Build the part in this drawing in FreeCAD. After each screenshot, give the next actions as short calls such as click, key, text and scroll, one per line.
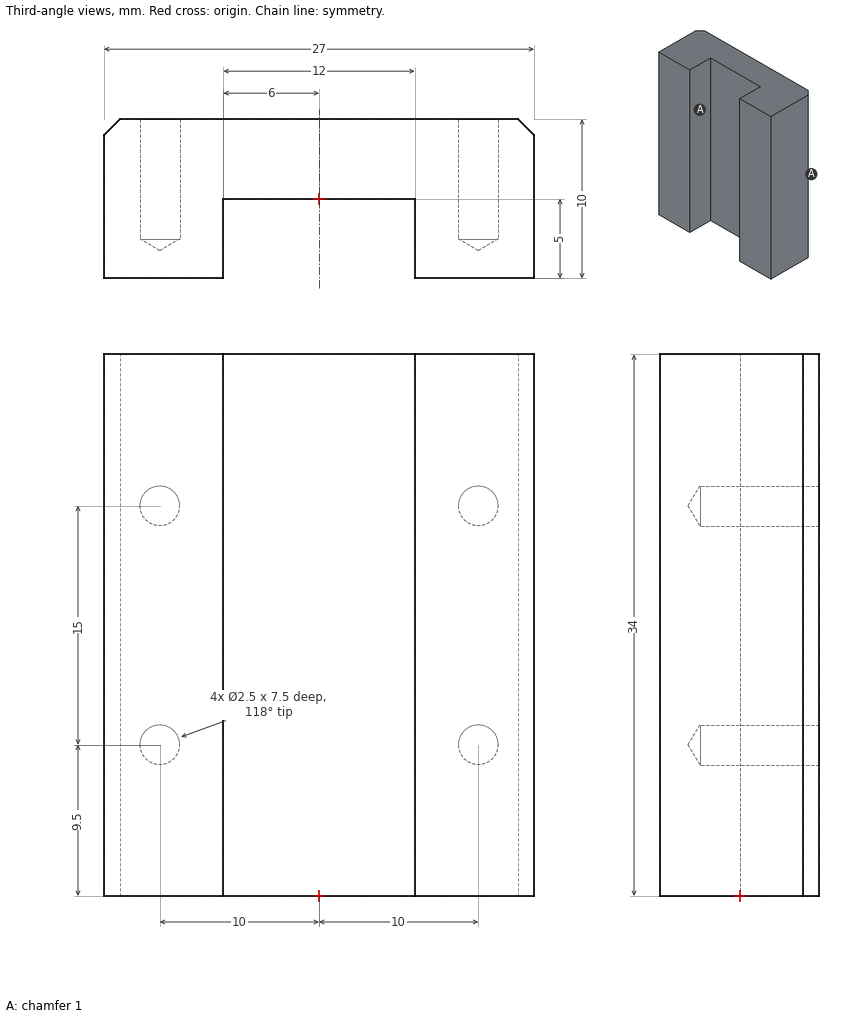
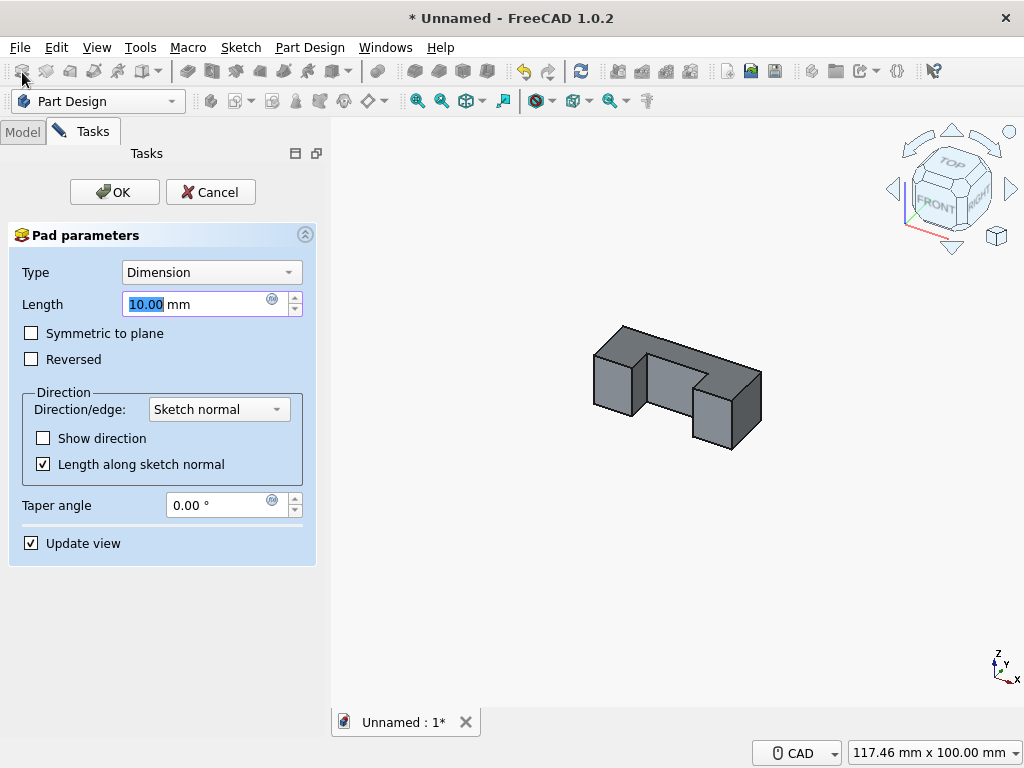
text(34)
key(Tab)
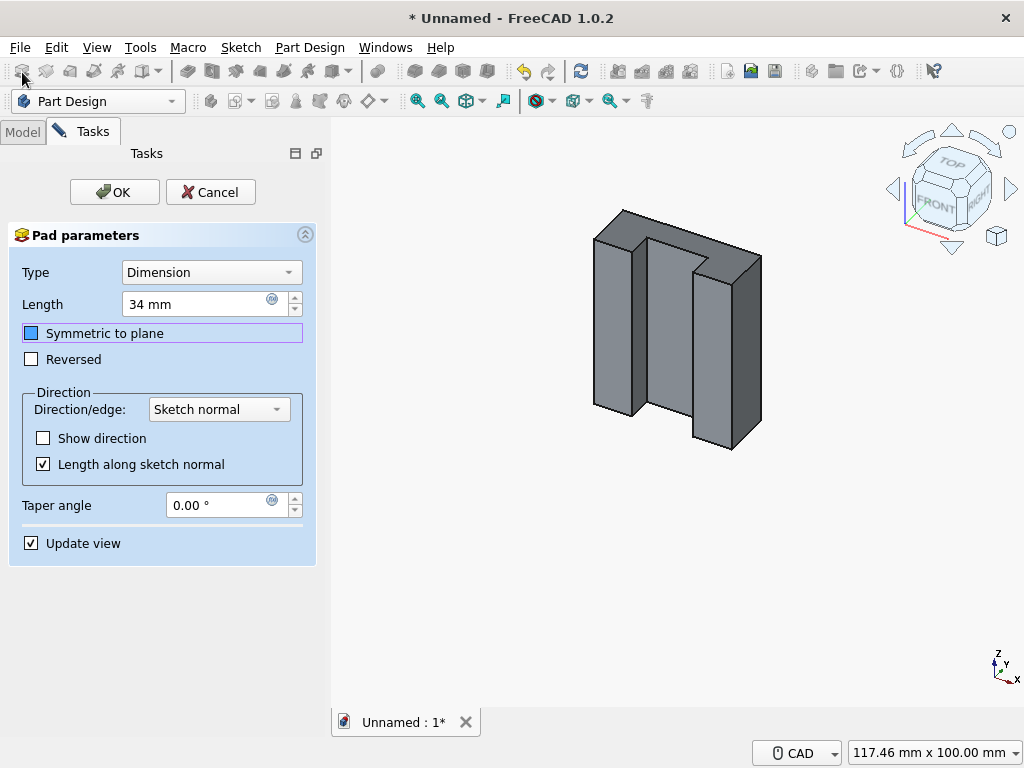
click(115, 192)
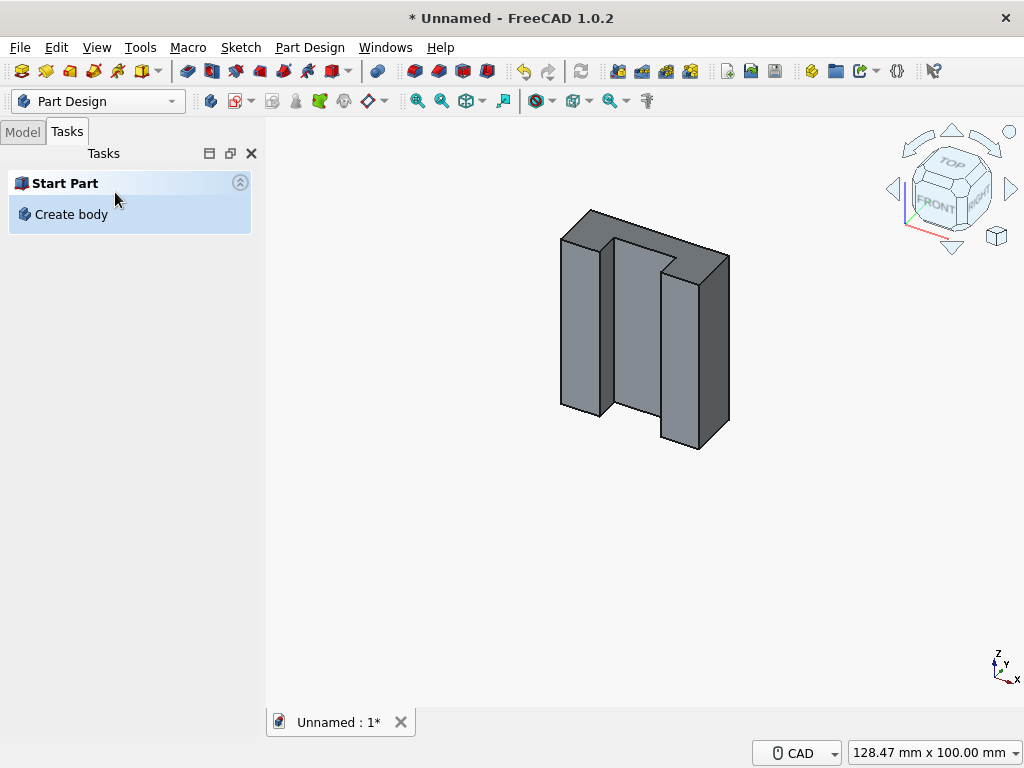
key(v)
key(f)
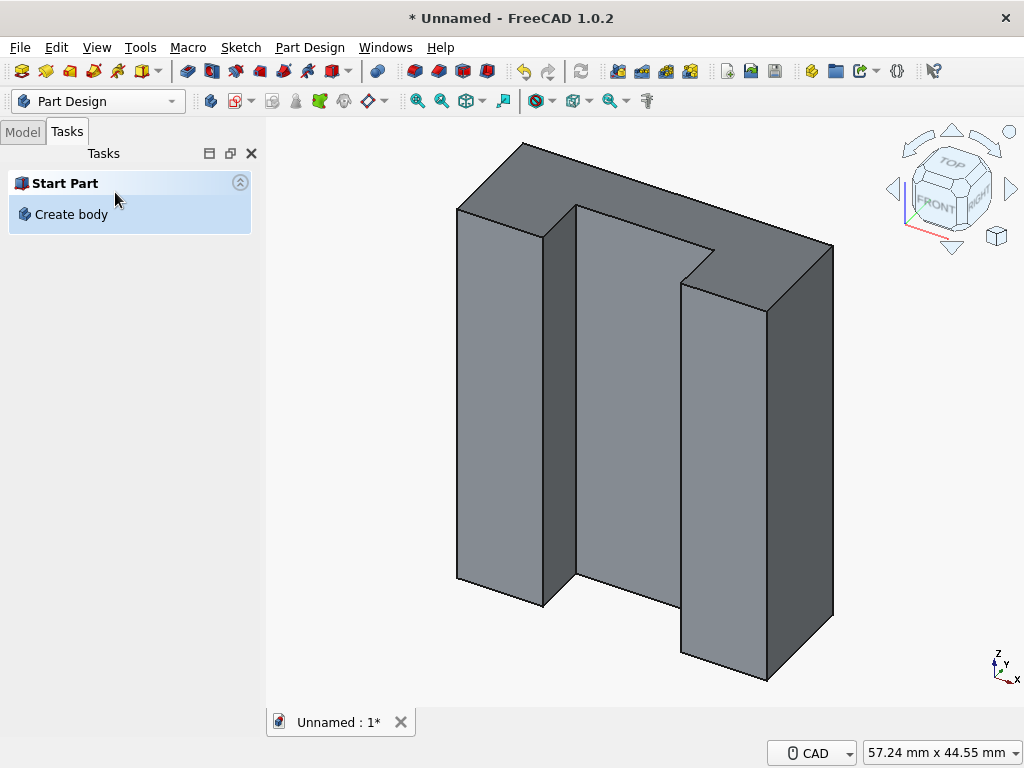
key(4)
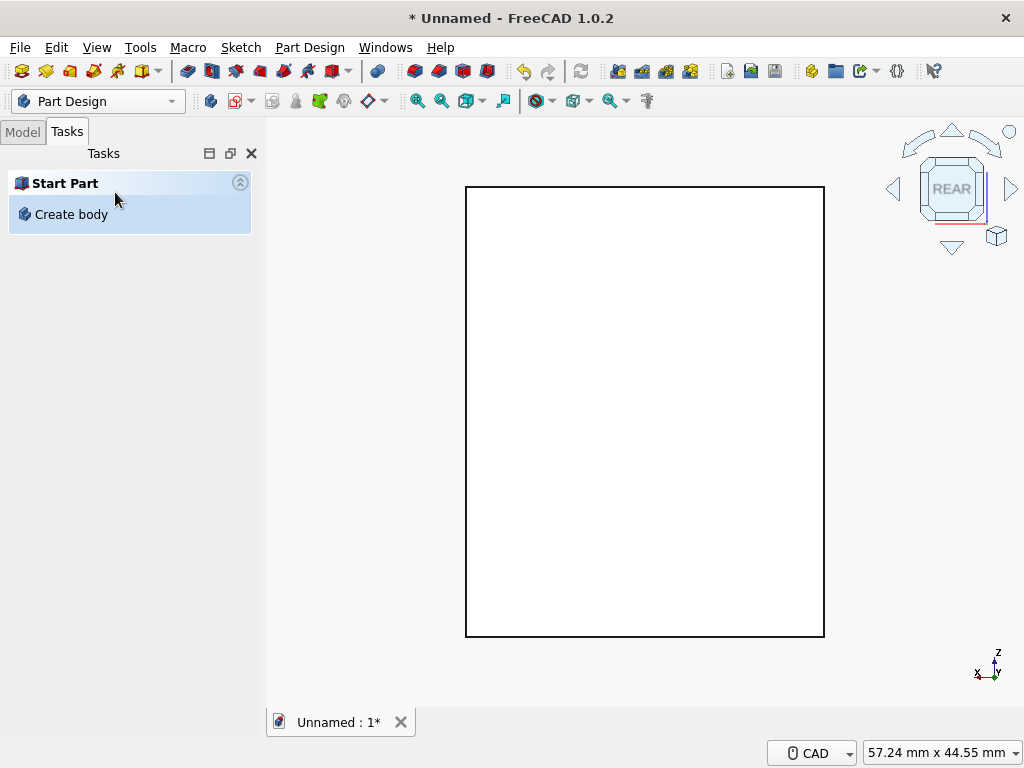
click(645, 411)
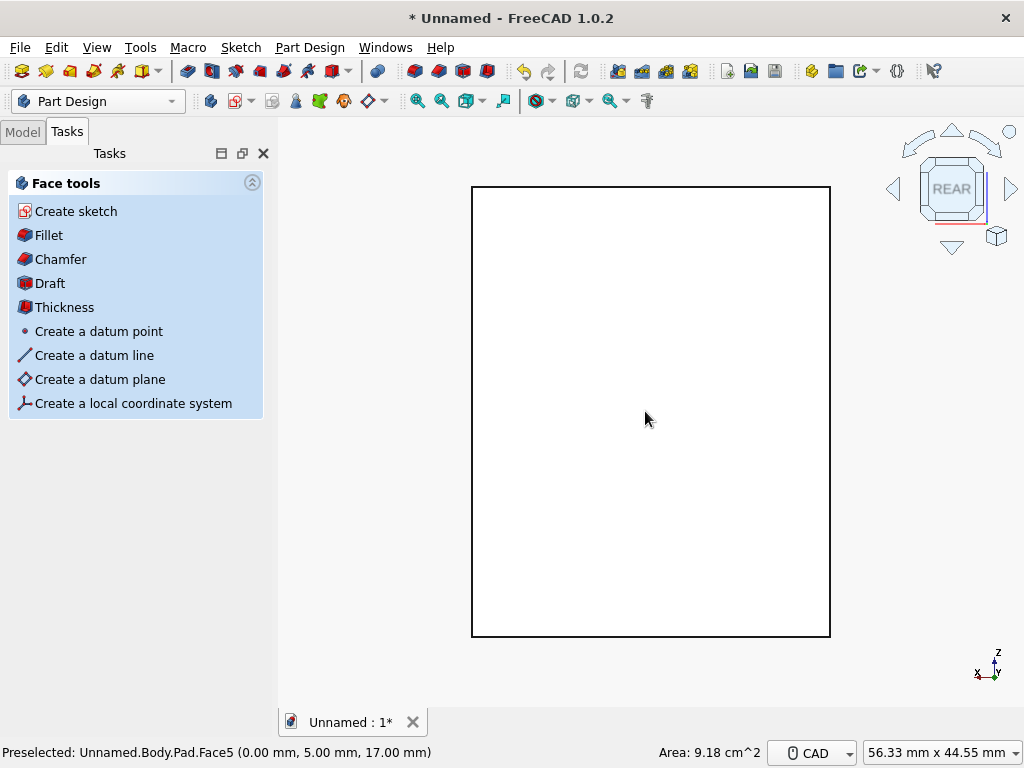
click(236, 102)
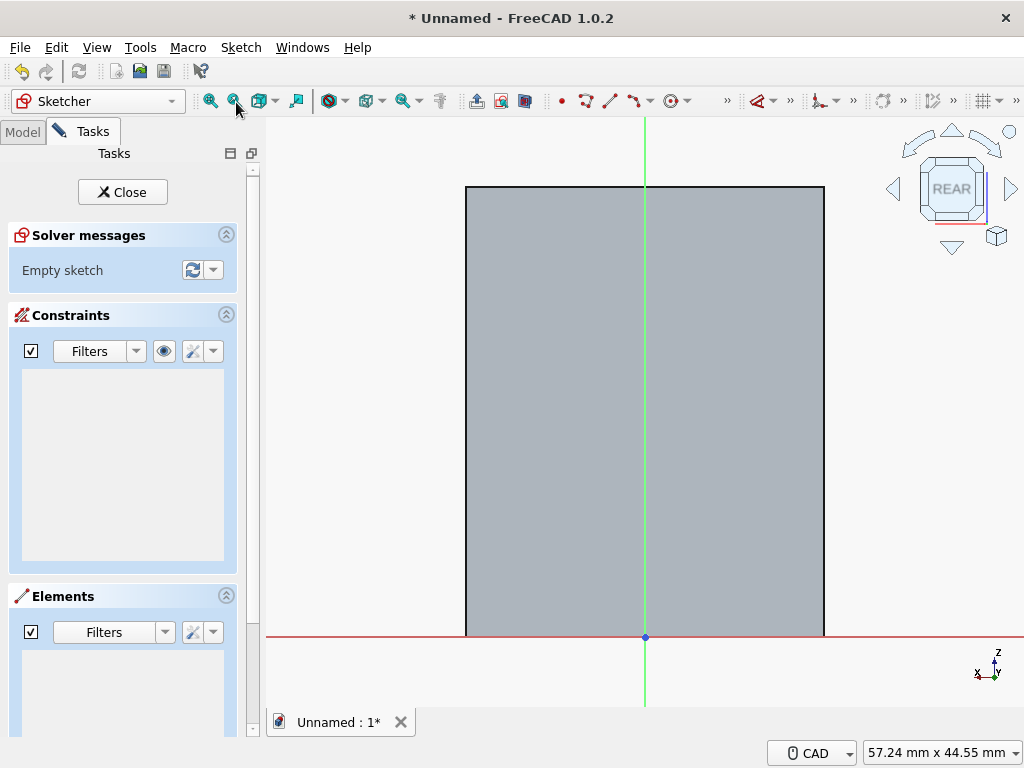
click(672, 102)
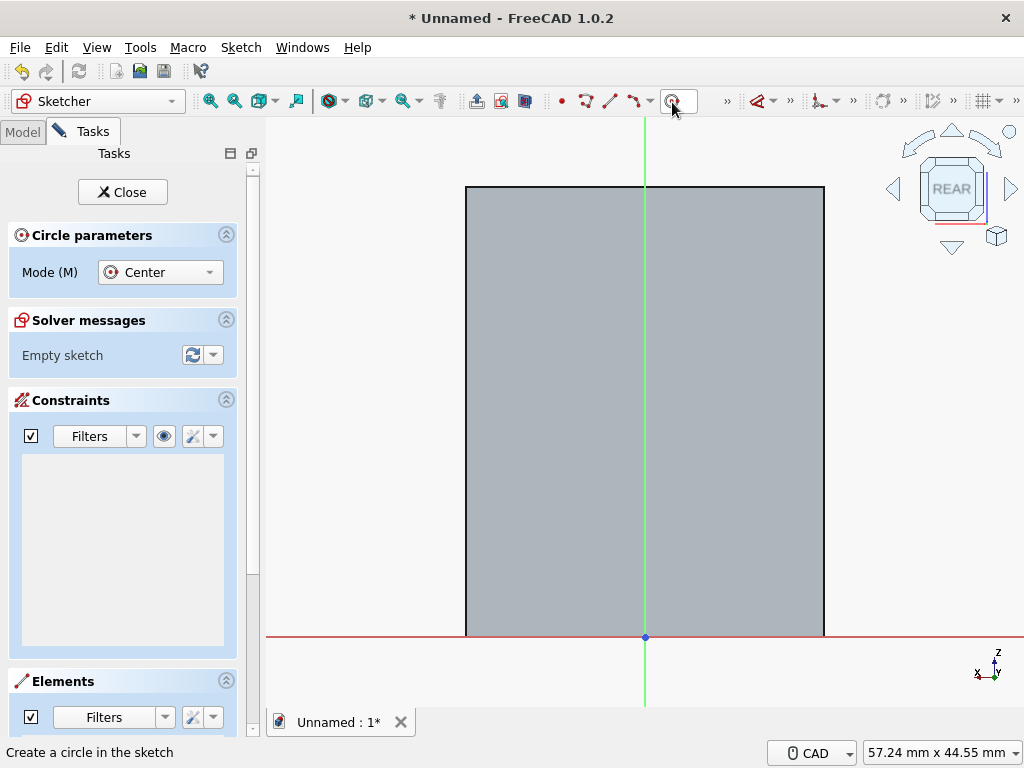
scroll(777, 511, up, 2)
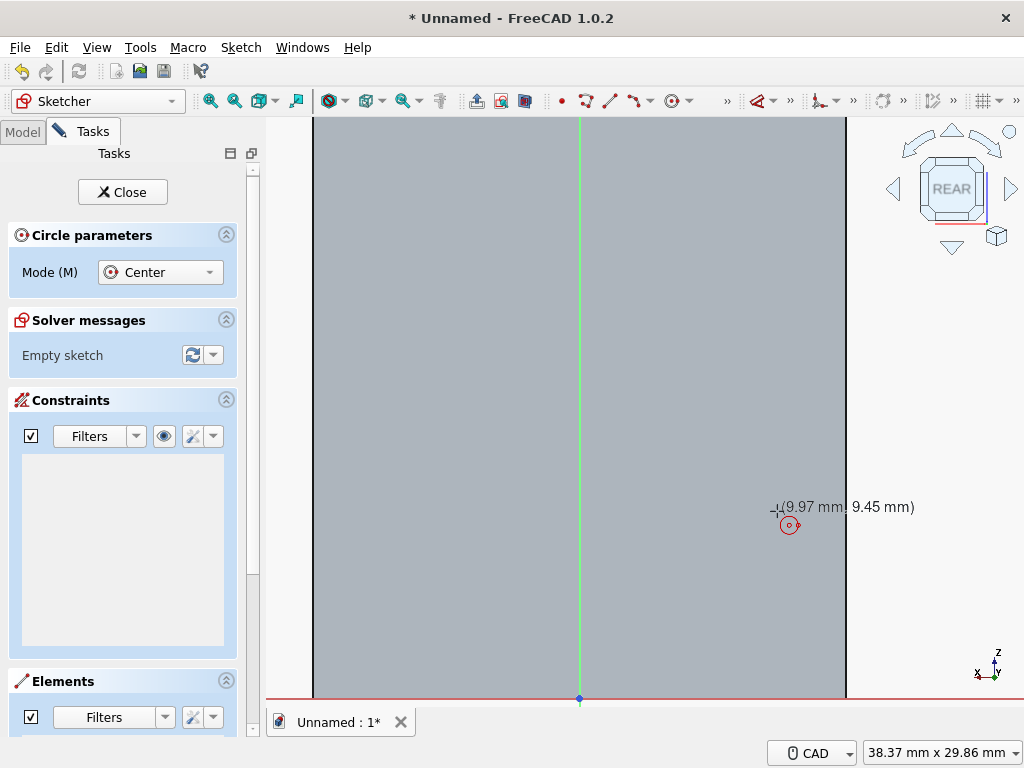
click(777, 511)
move(795, 494)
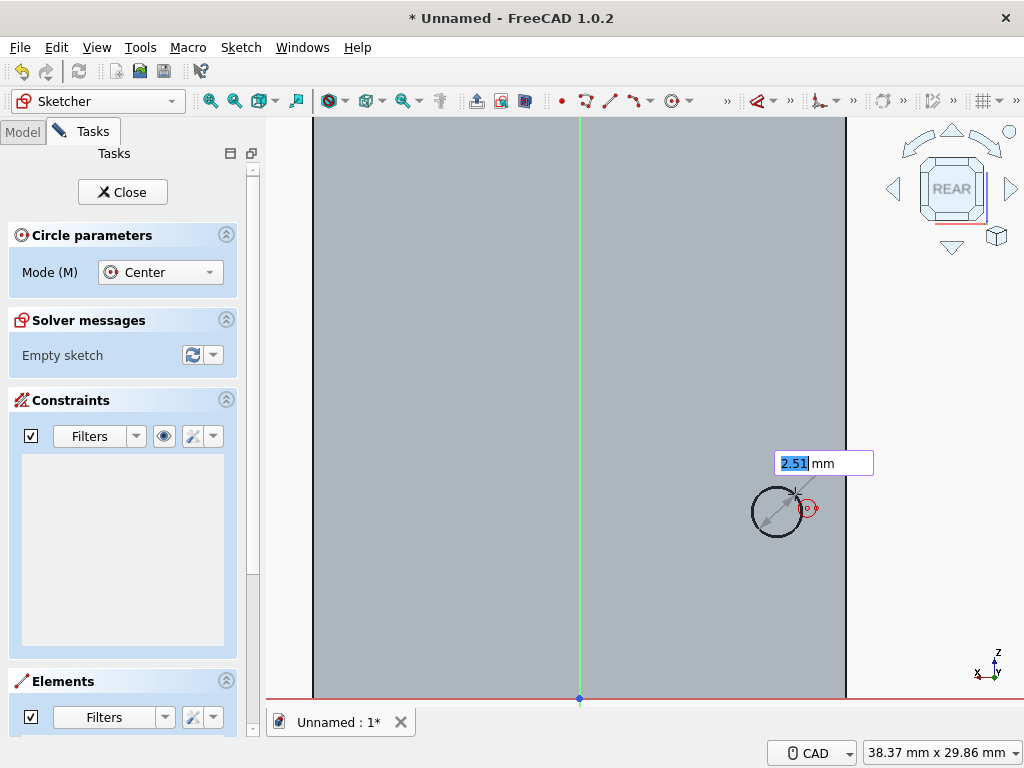
text(2.5)
key(Return)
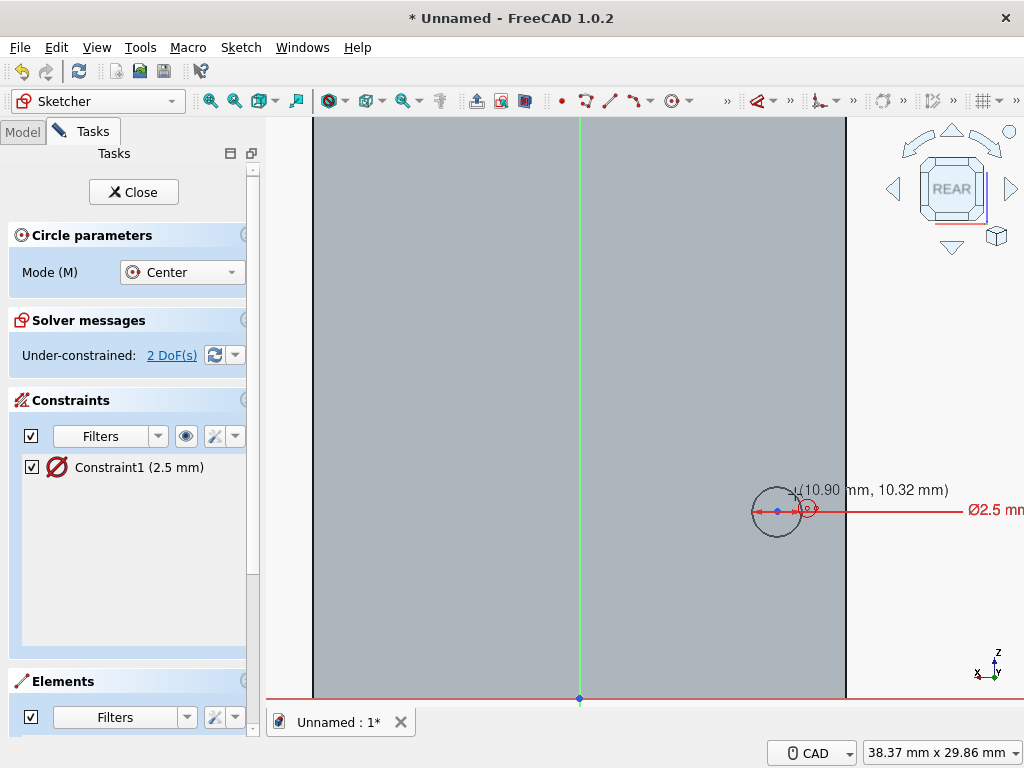
click(382, 511)
move(400, 494)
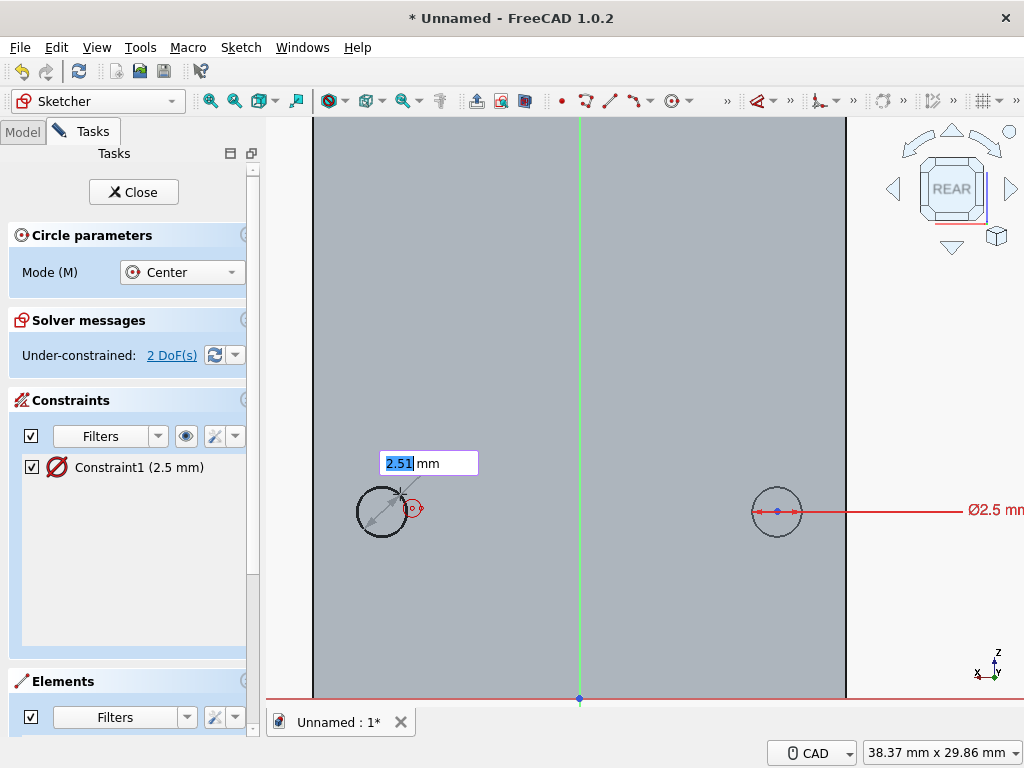
text(2.5)
key(Return)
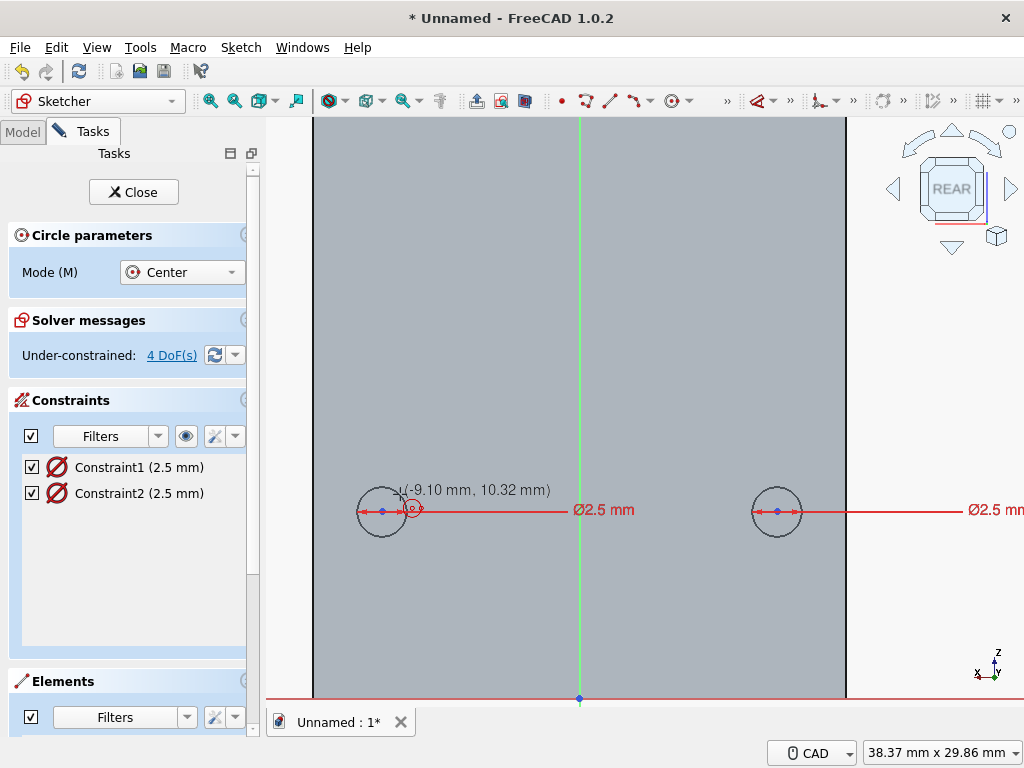
click(777, 215)
move(795, 197)